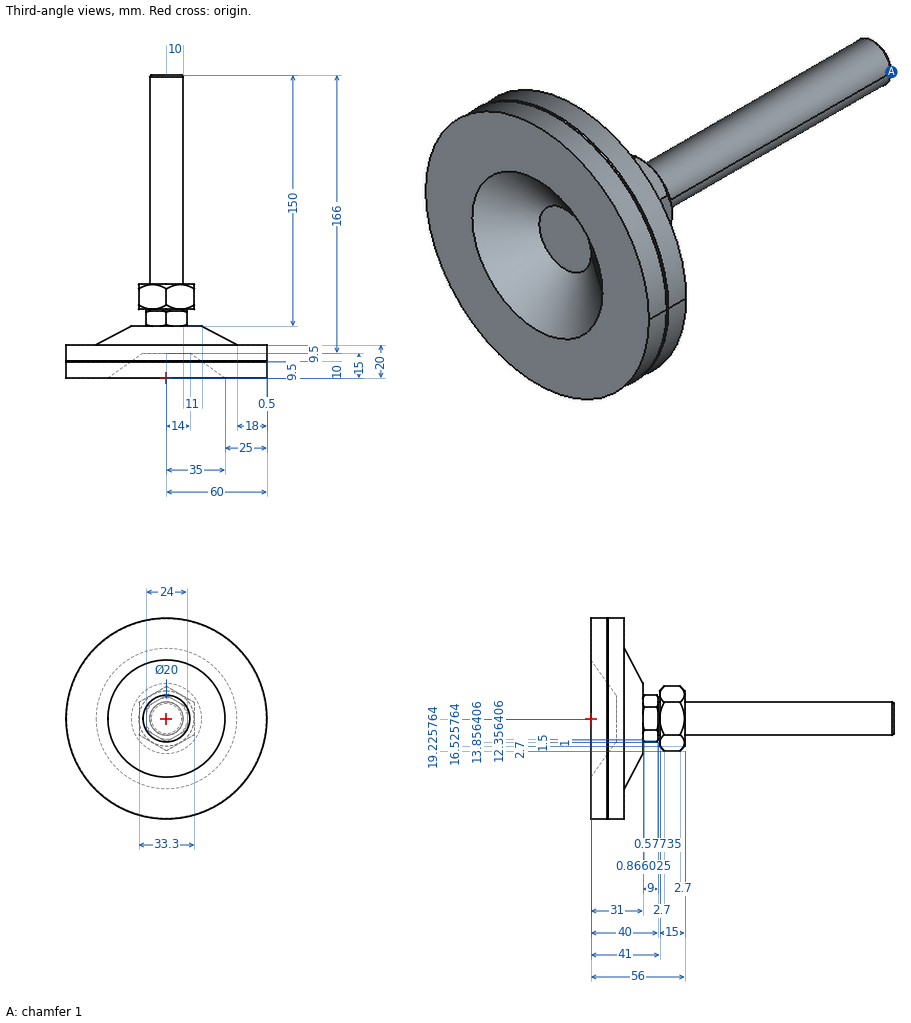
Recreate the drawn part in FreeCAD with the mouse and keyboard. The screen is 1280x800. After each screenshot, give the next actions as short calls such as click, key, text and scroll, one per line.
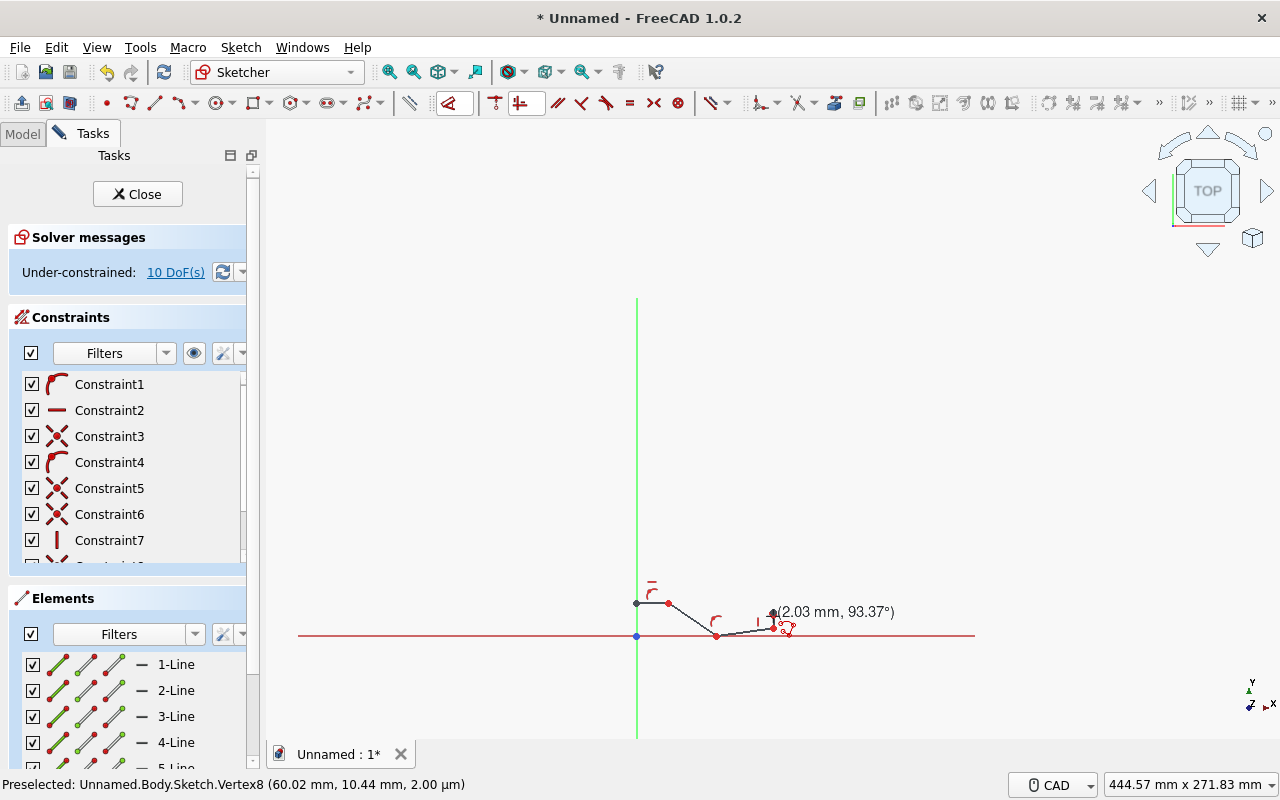
click(774, 590)
click(733, 590)
click(685, 565)
click(660, 565)
click(660, 223)
click(646, 223)
click(637, 603)
key(Escape)
key(Escape)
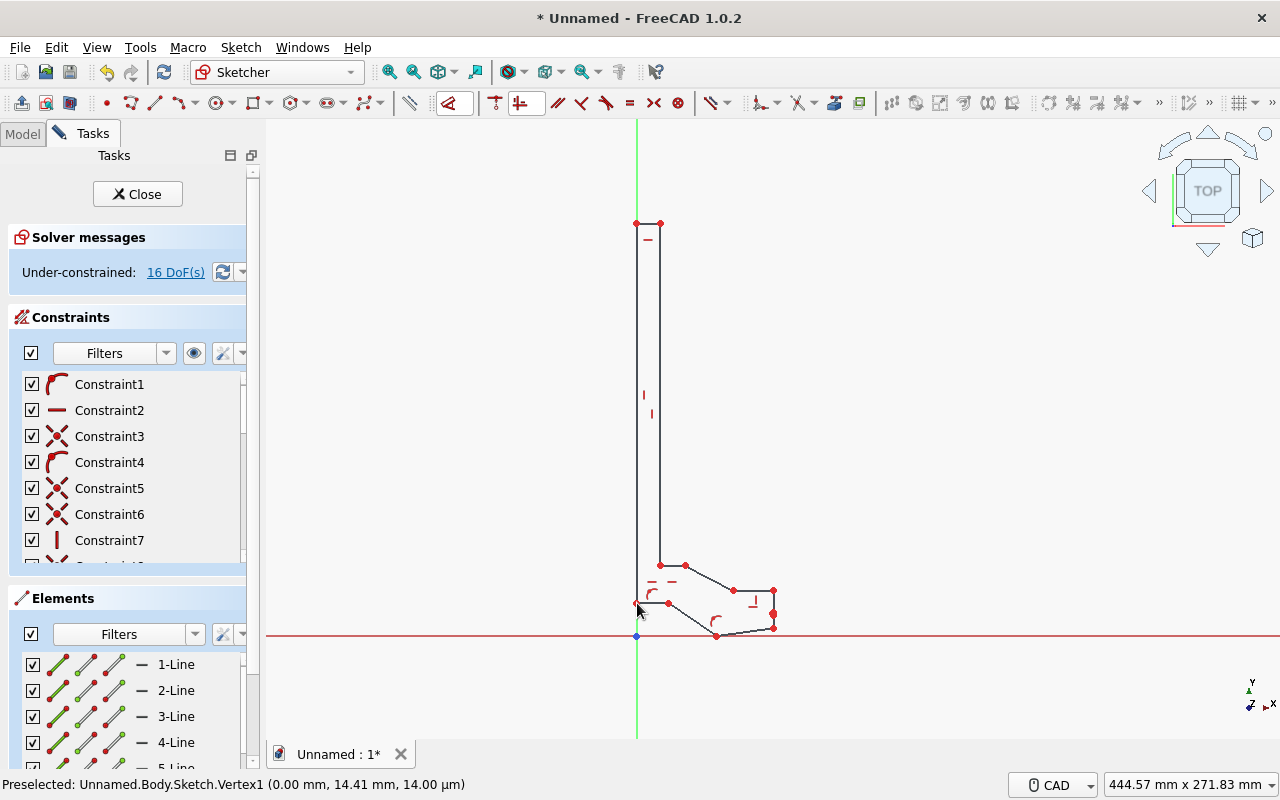
click(734, 634)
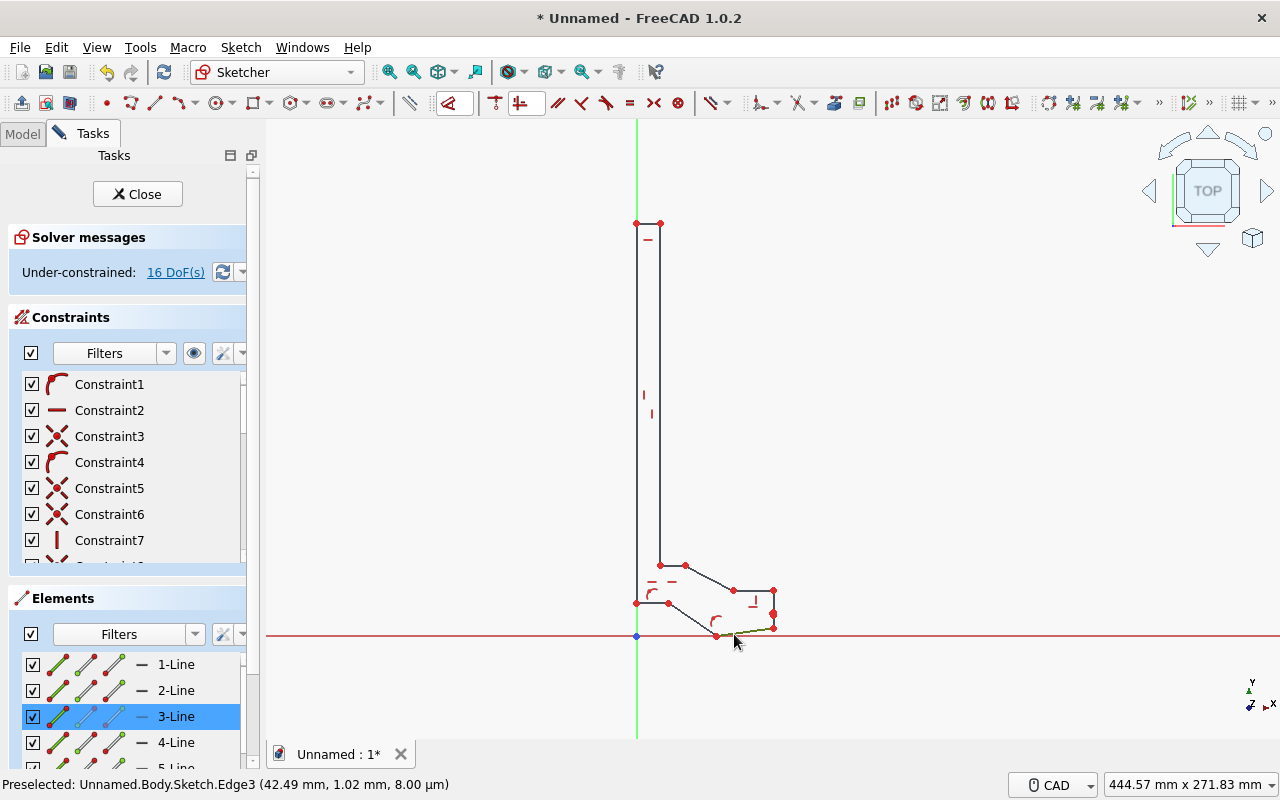
key(h)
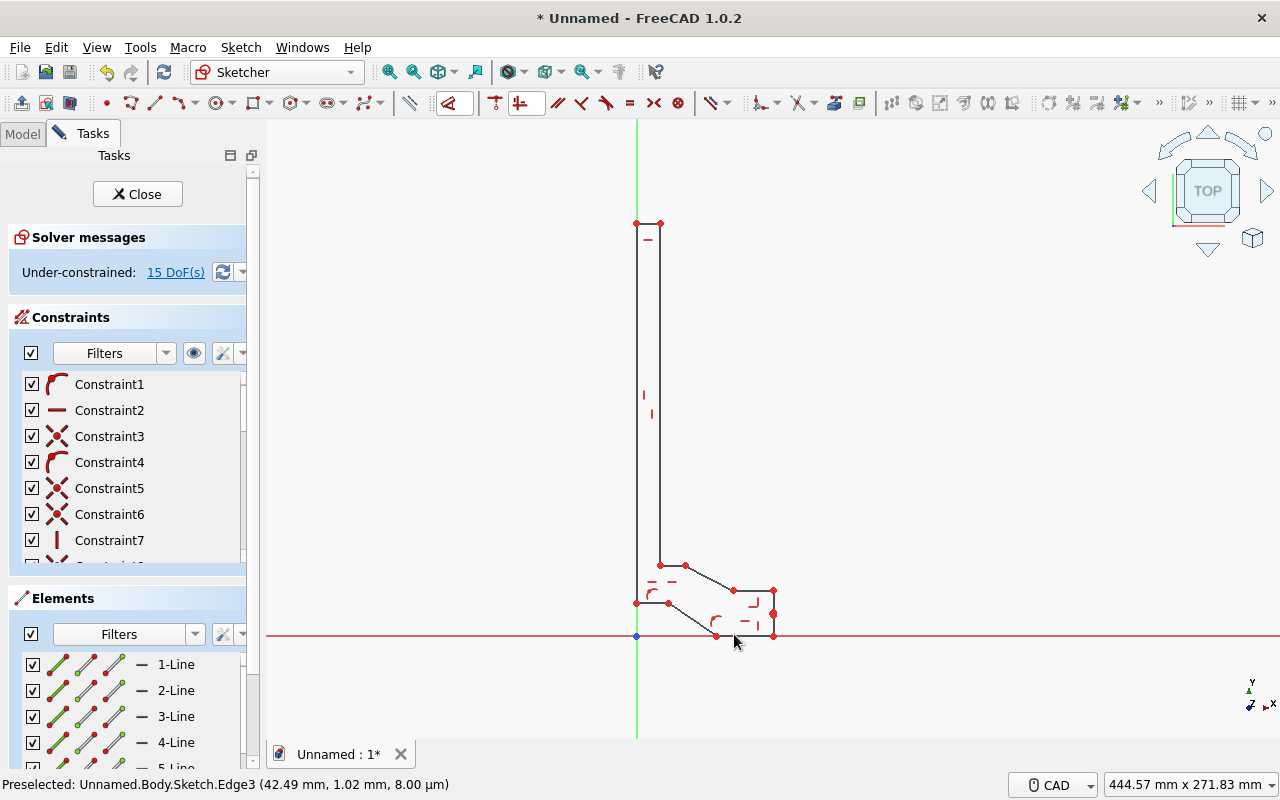
click(448, 104)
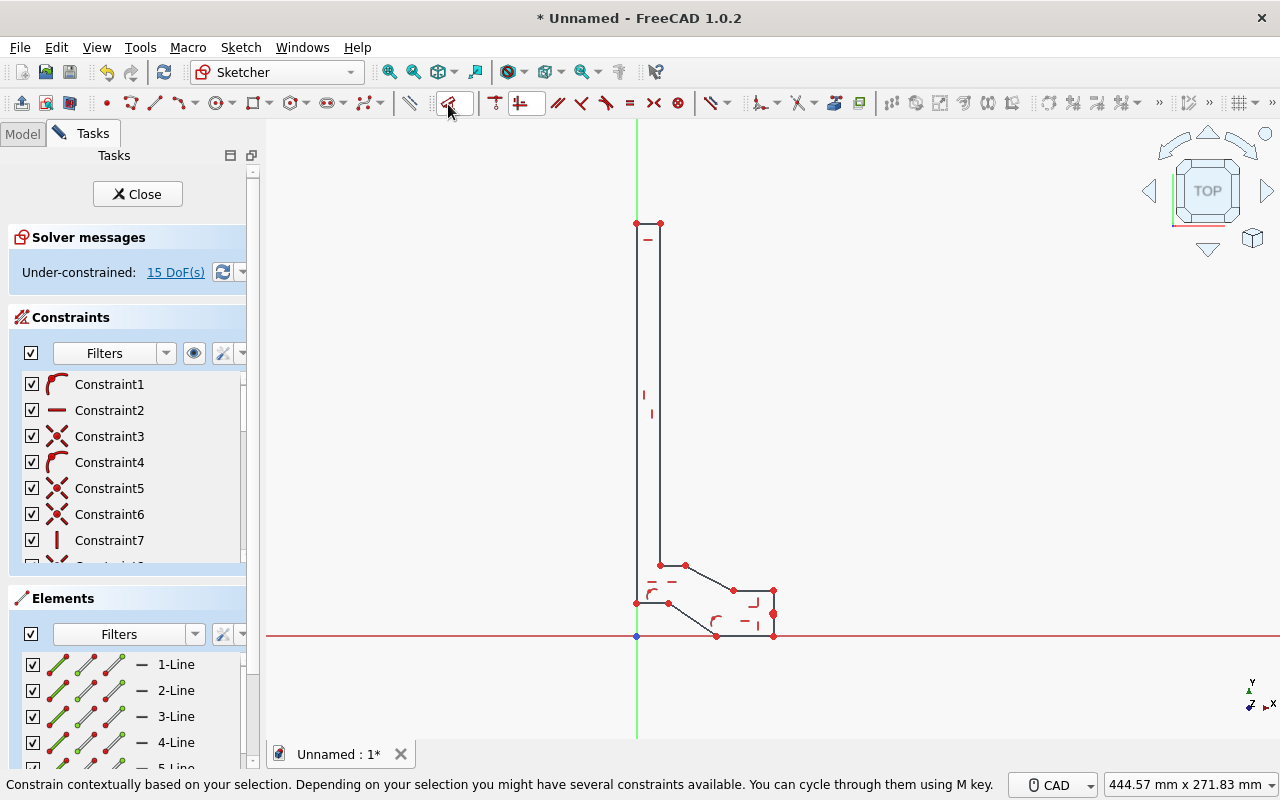
scroll(647, 603, up, 2)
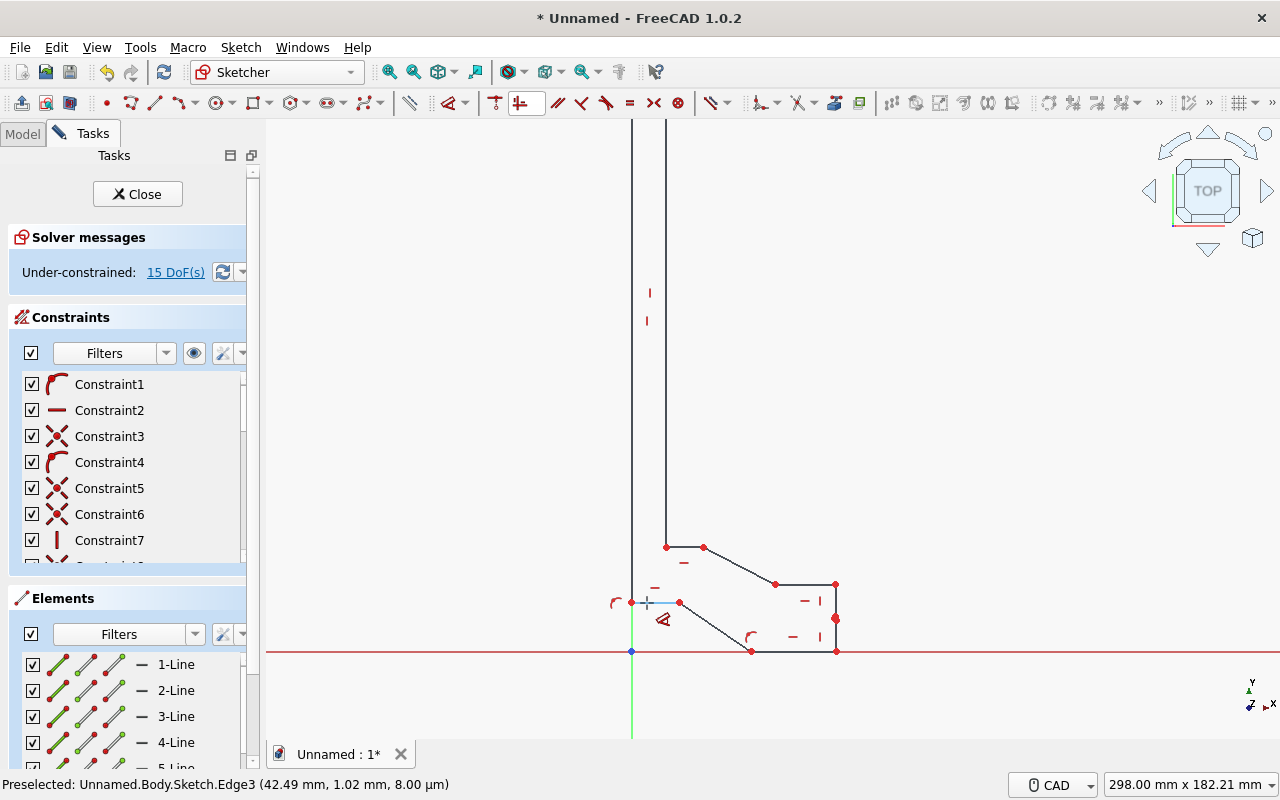
click(646, 603)
click(656, 637)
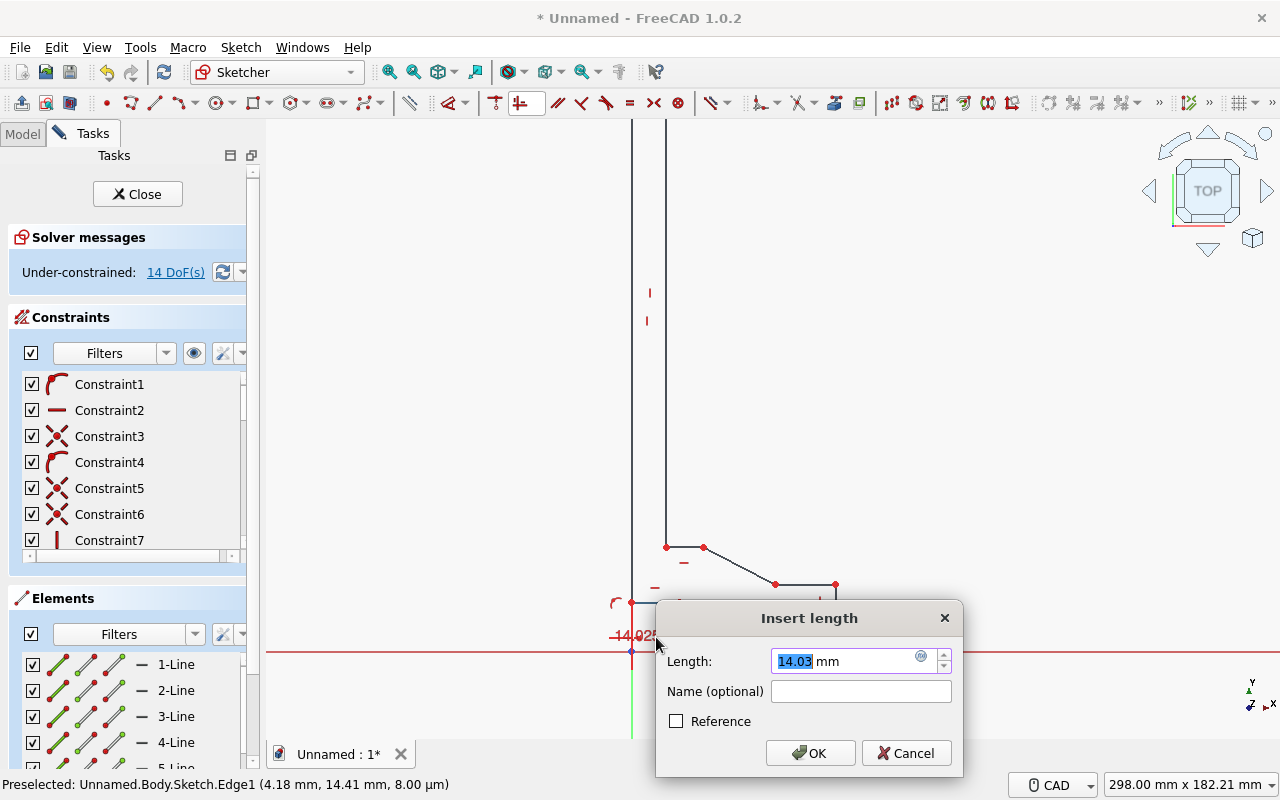
text(14)
key(Return)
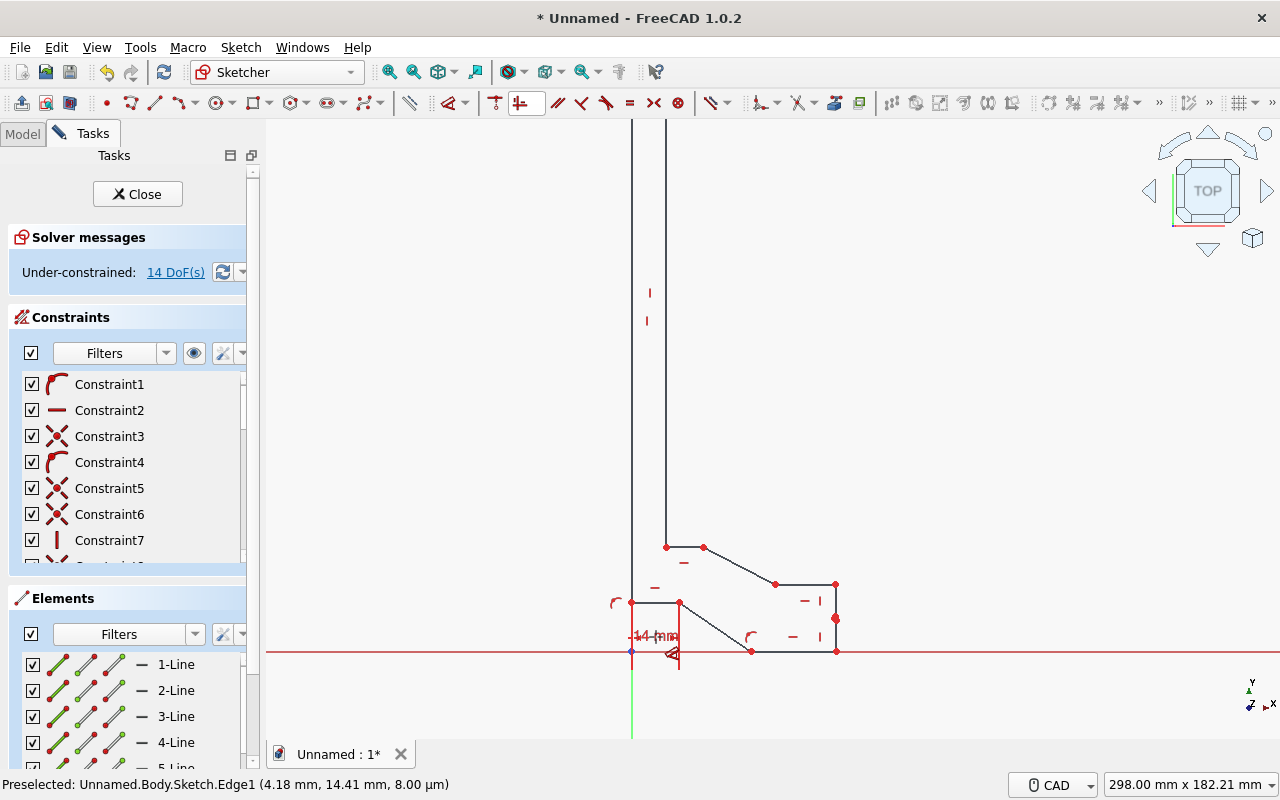
click(777, 652)
click(794, 686)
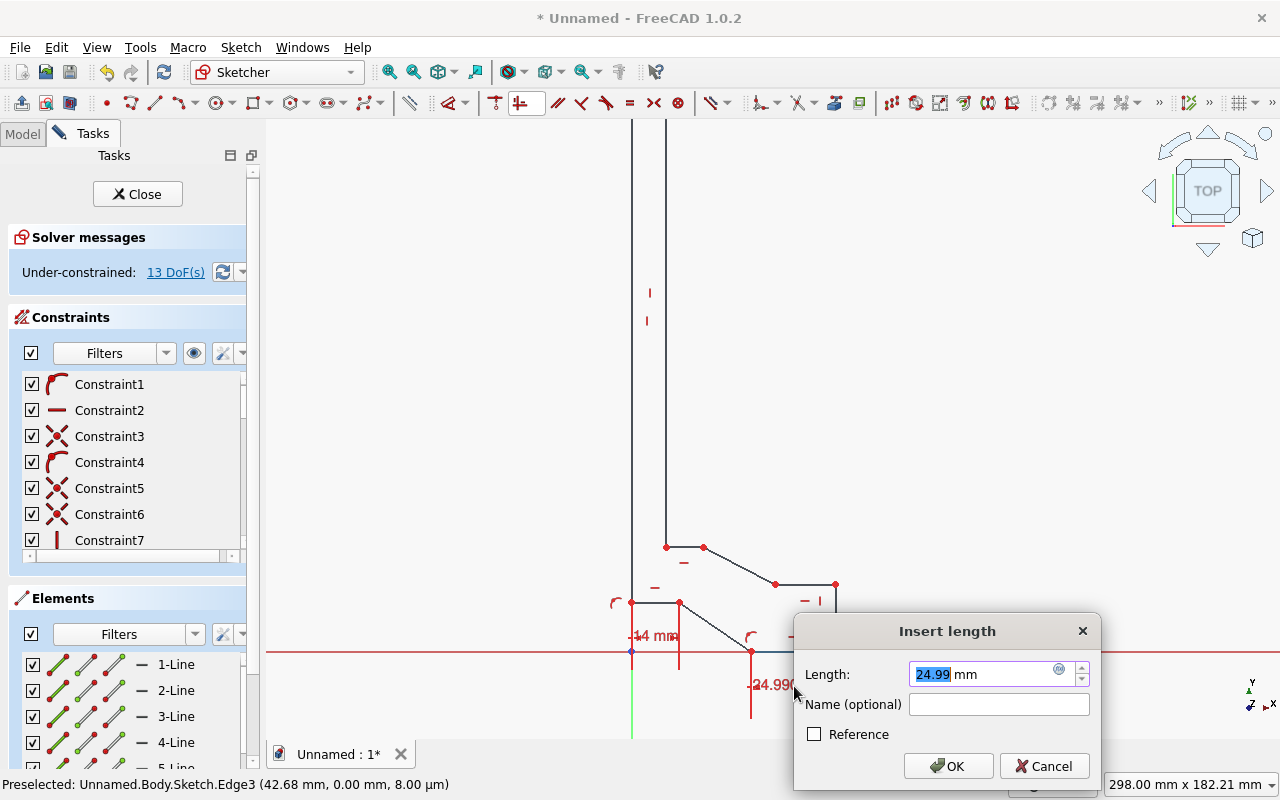
text(25)
key(Return)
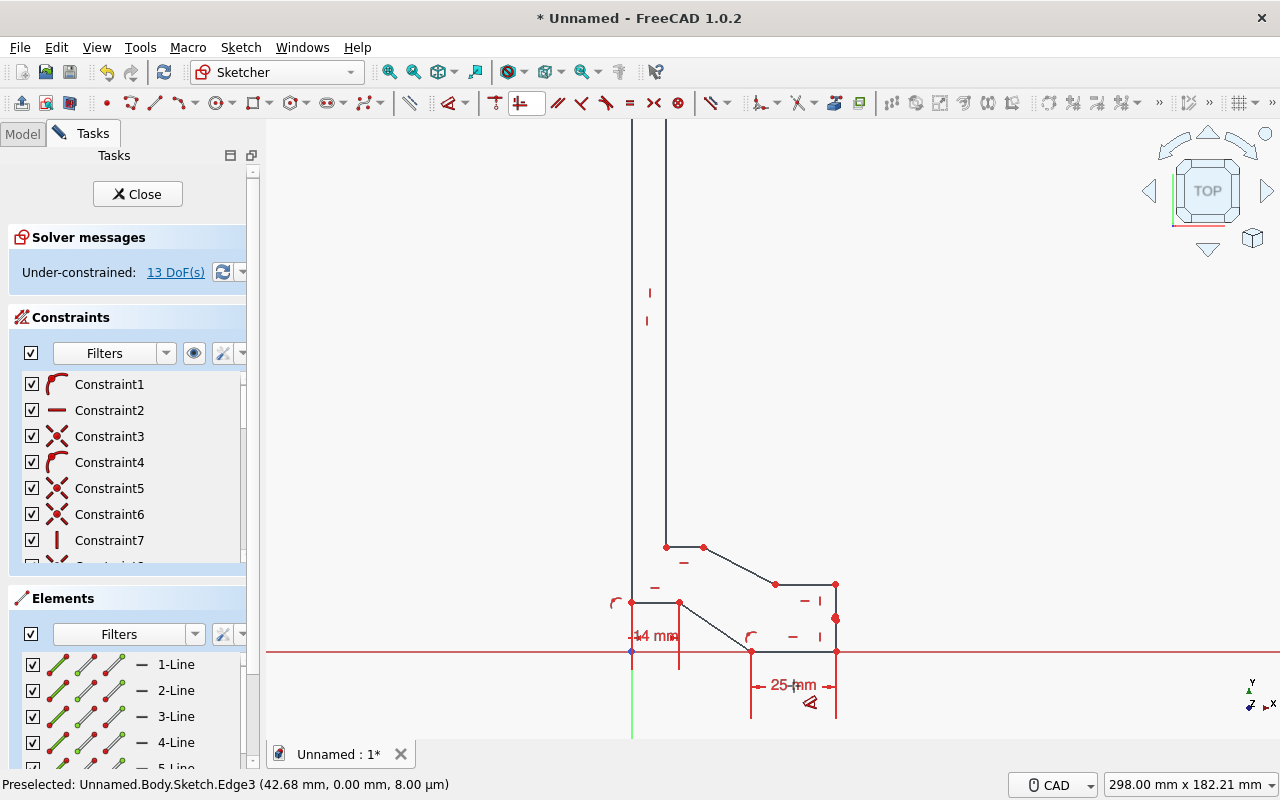
click(818, 585)
click(805, 619)